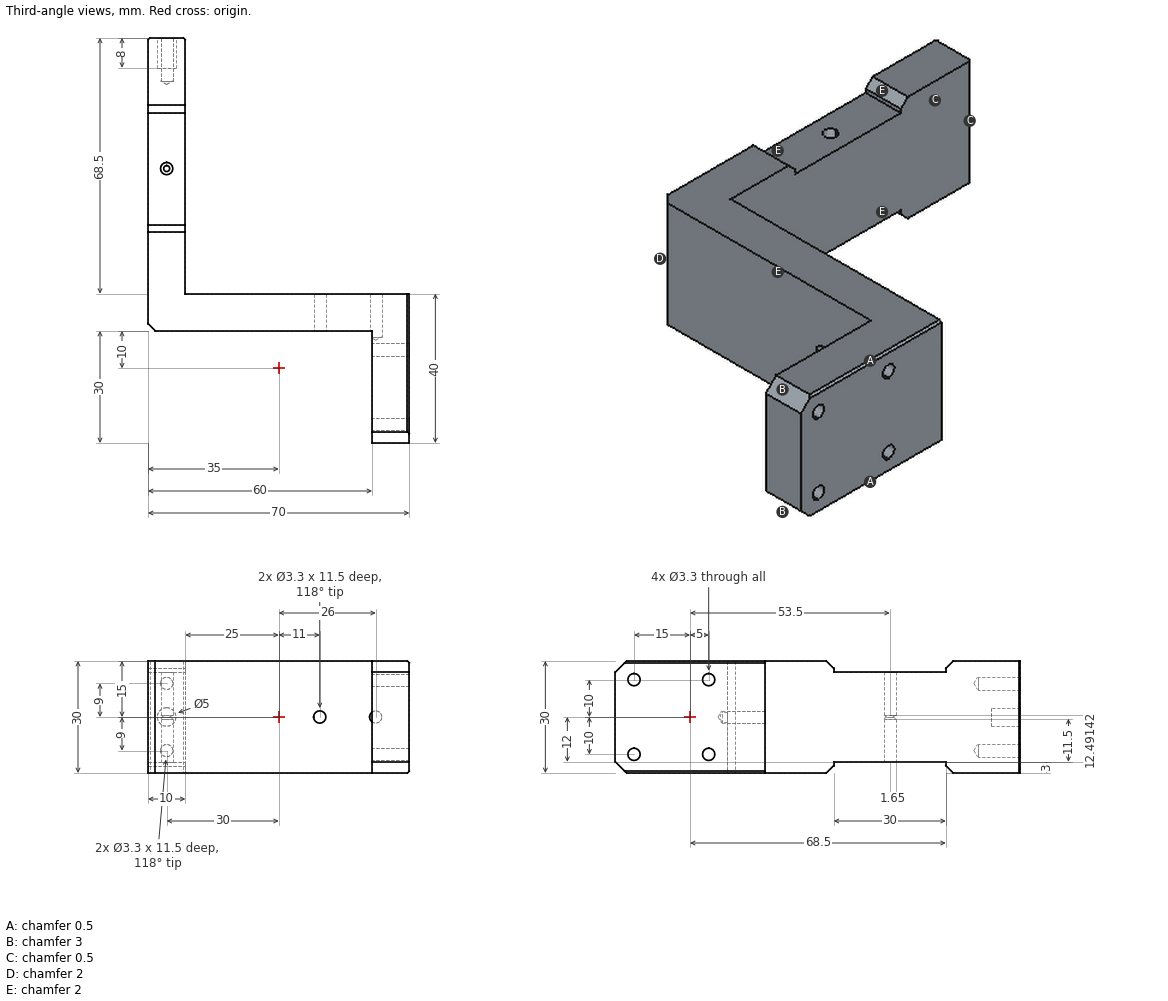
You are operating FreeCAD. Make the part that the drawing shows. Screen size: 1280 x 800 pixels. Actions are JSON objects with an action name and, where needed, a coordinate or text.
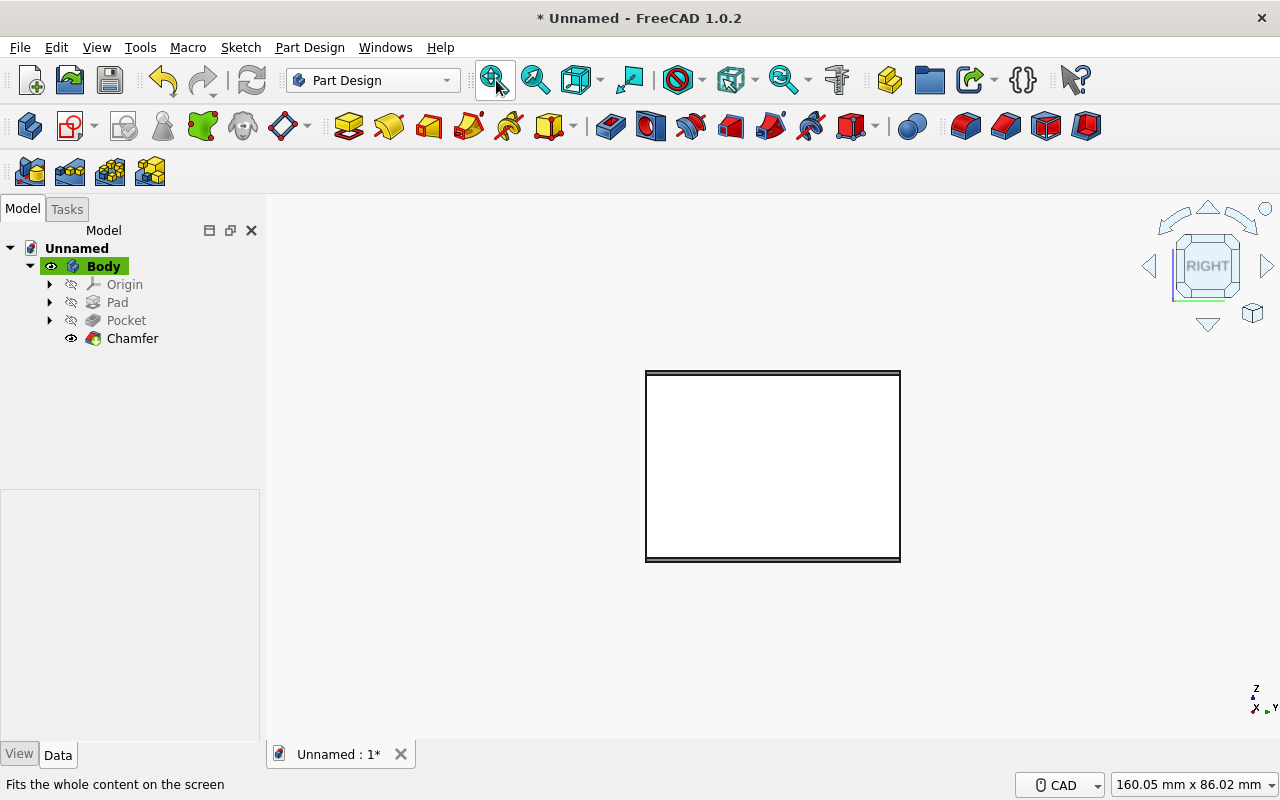
{"action": "key", "text": "v f"}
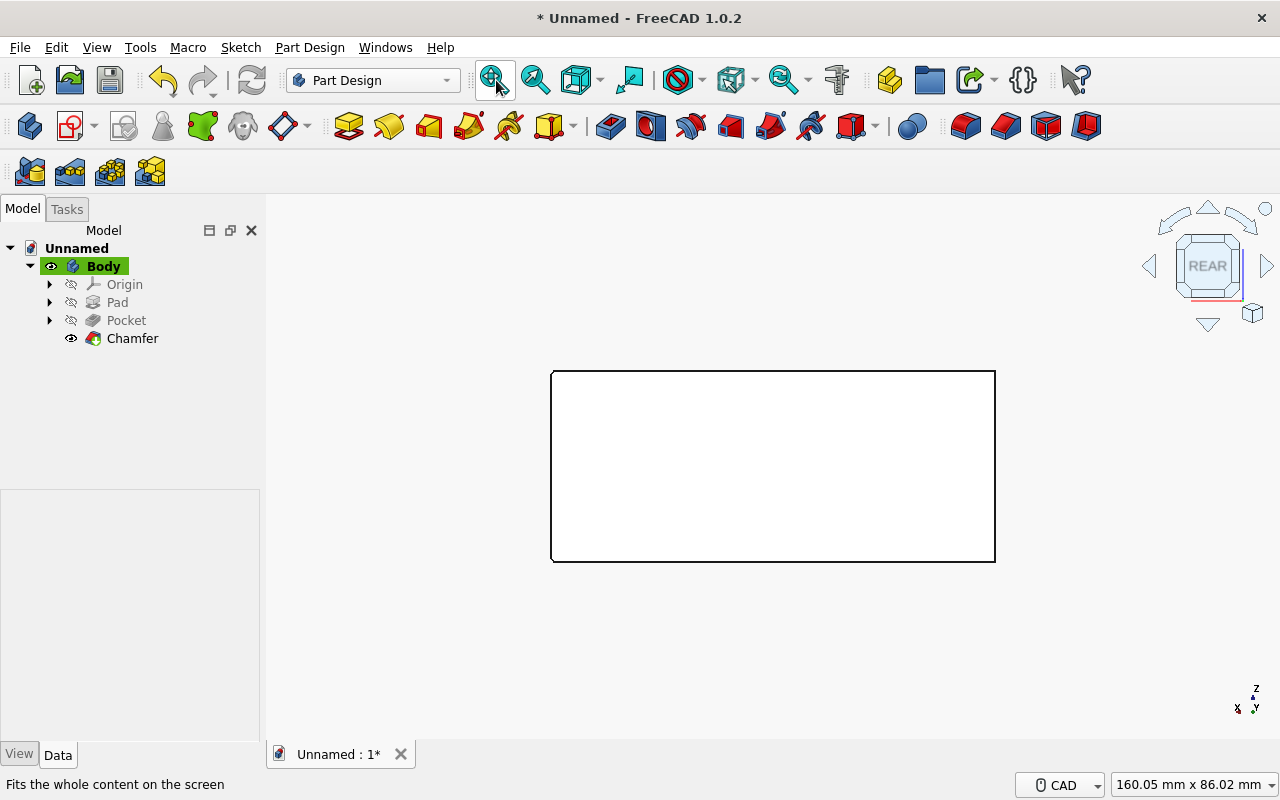
{"action": "left_click", "coordinate": [646, 466]}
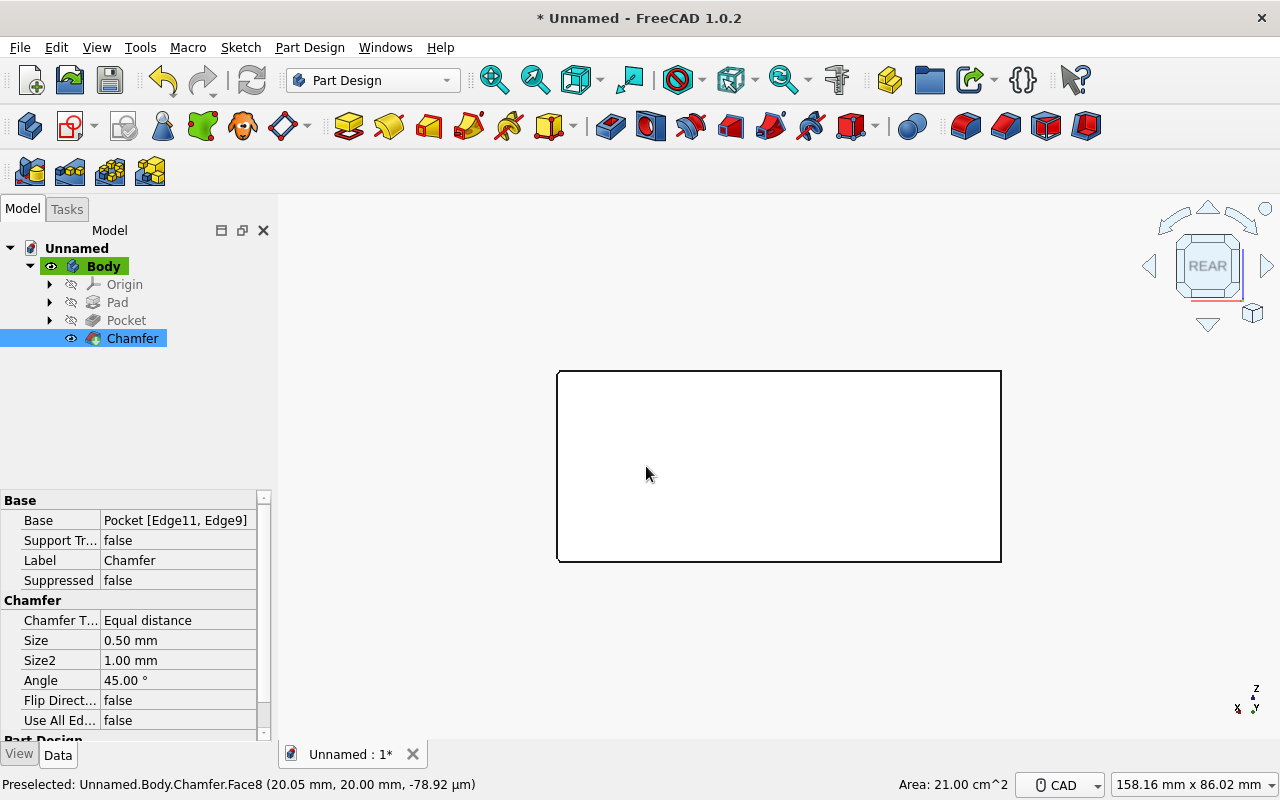
{"action": "left_click", "coordinate": [70, 126]}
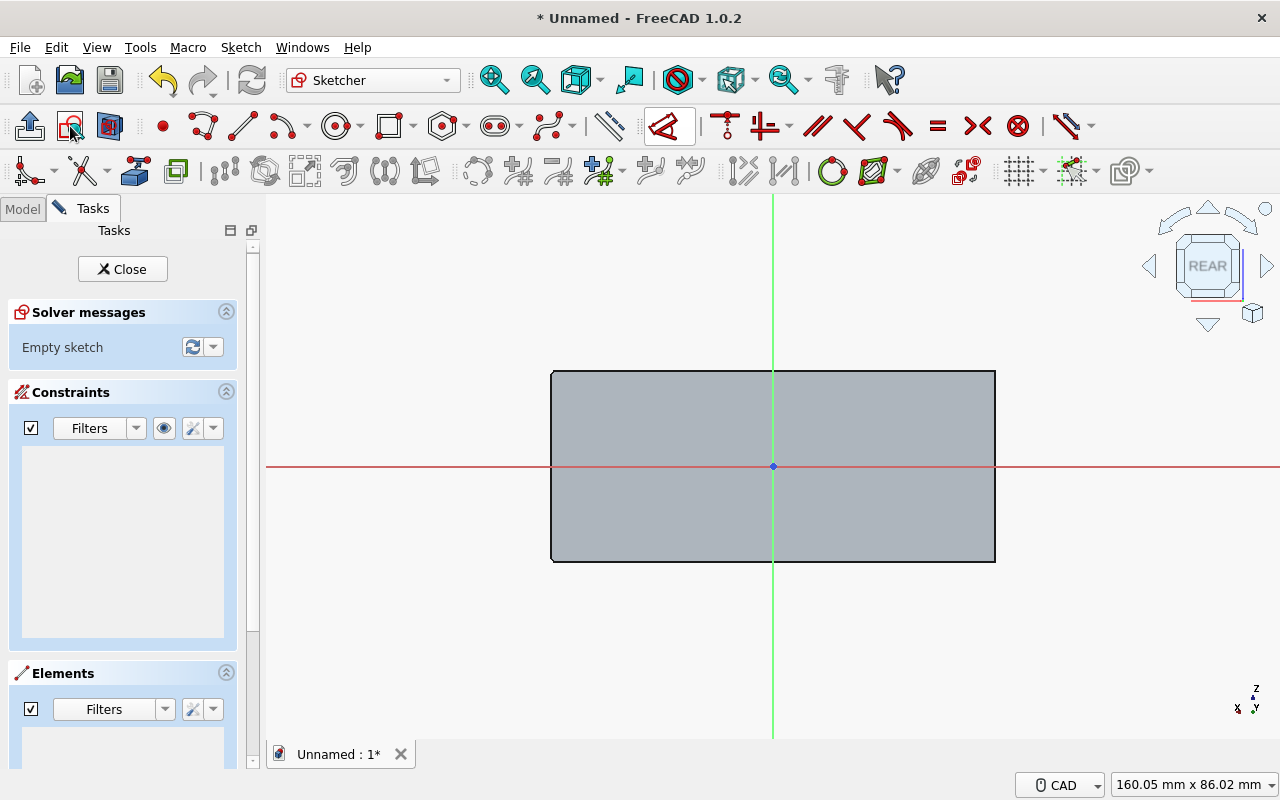
{"action": "scroll", "coordinate": [677, 466], "scroll_direction": "up", "scroll_amount": 6}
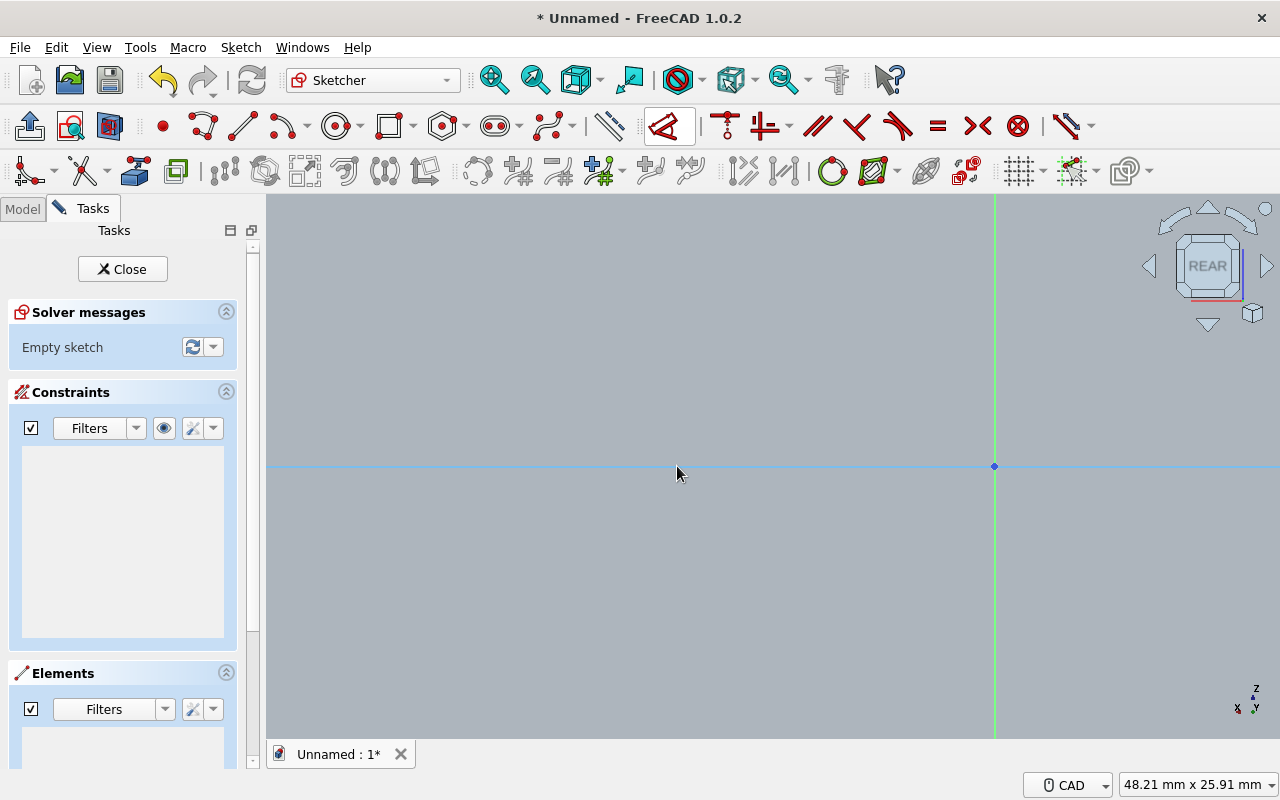
{"action": "key", "text": "g c"}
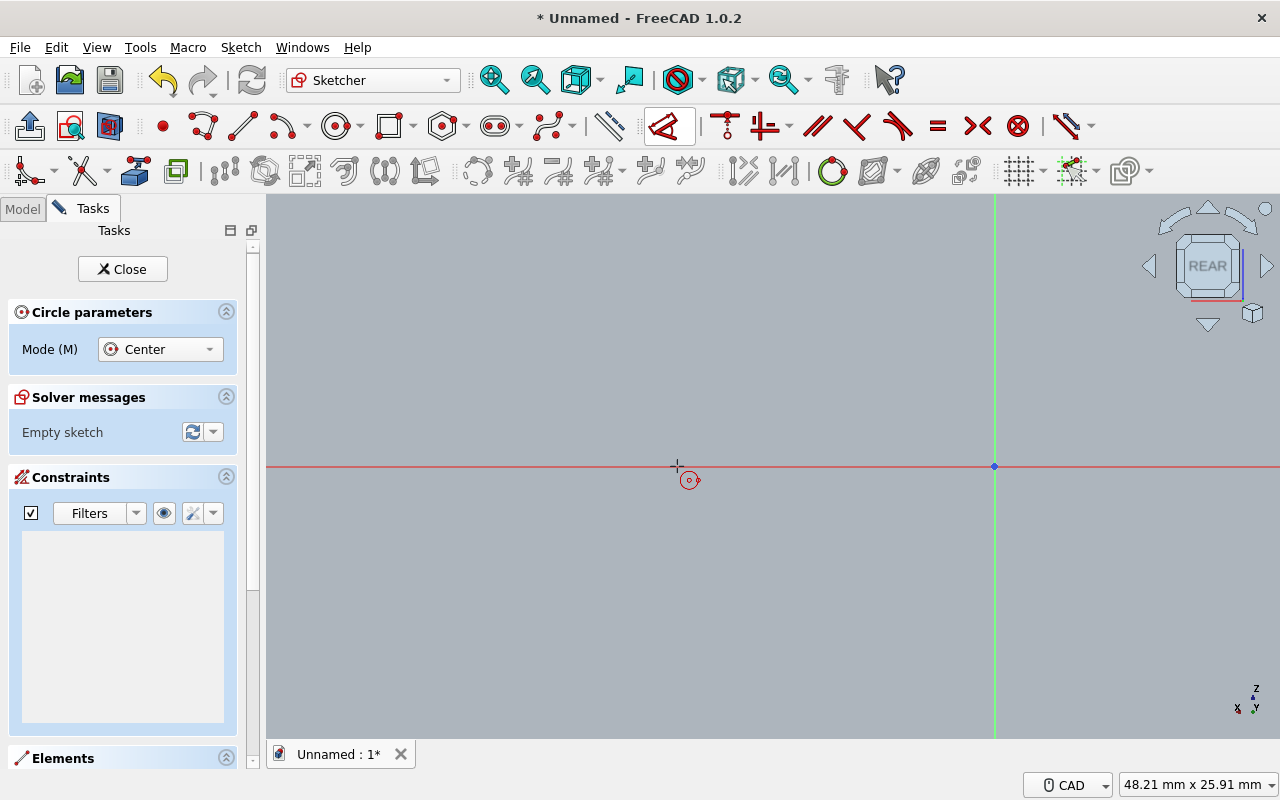
{"action": "left_click", "coordinate": [763, 466]}
{"action": "left_click", "coordinate": [788, 442]}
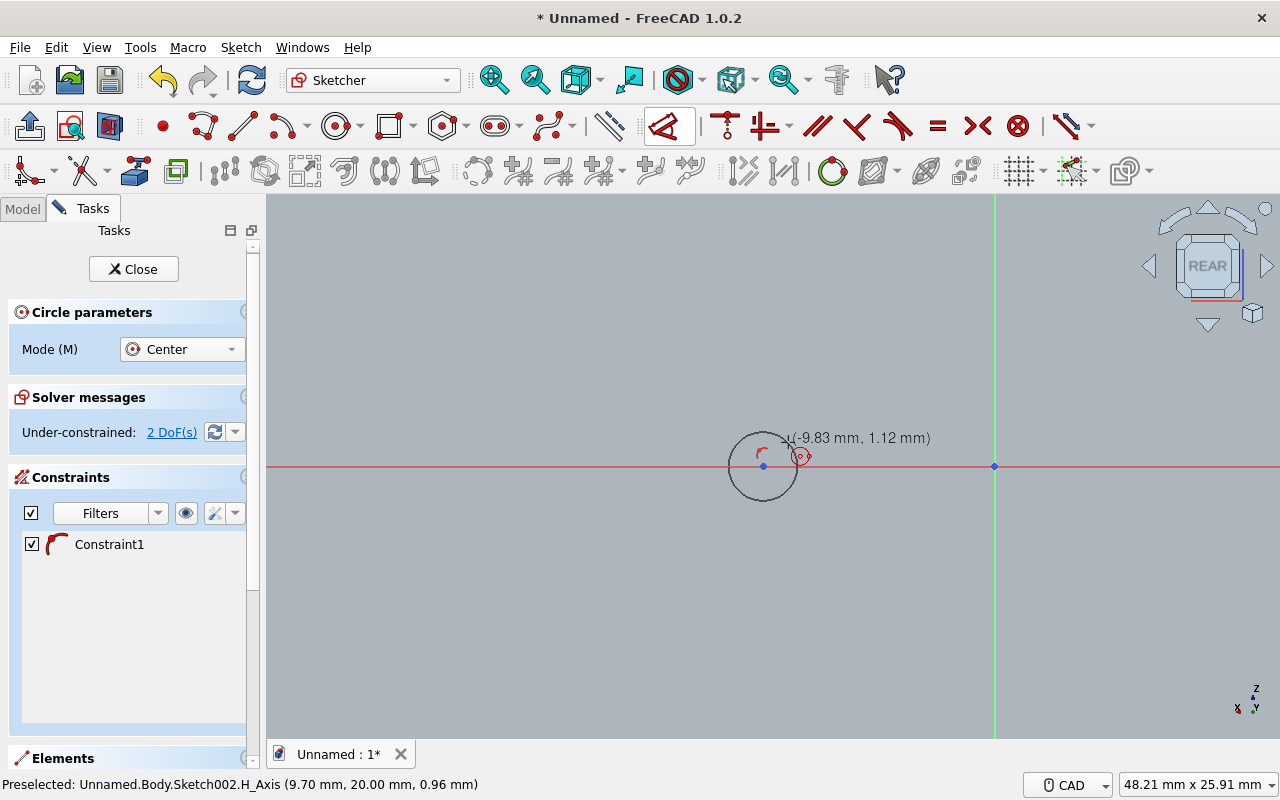
{"action": "left_click", "coordinate": [448, 466]}
{"action": "left_click", "coordinate": [472, 442]}
{"action": "key", "text": "Escape"}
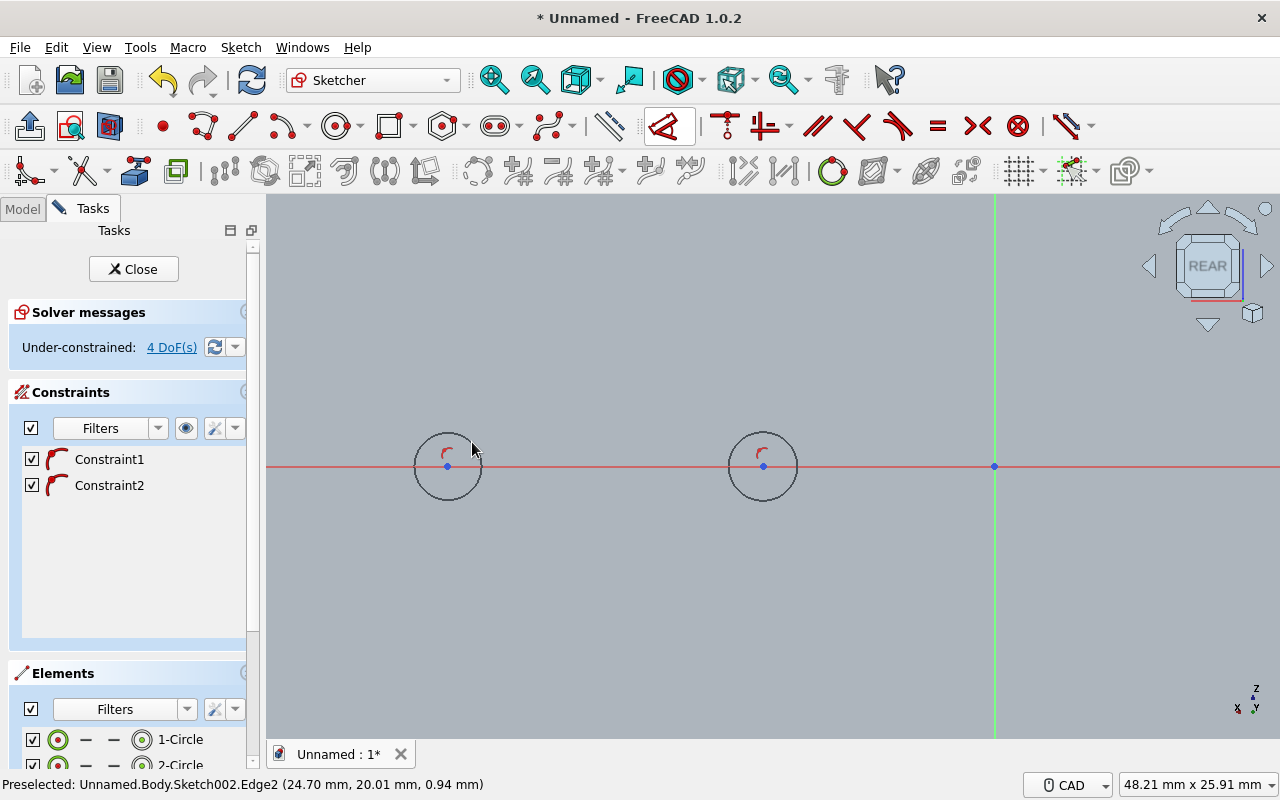
{"action": "left_click", "coordinate": [787, 442]}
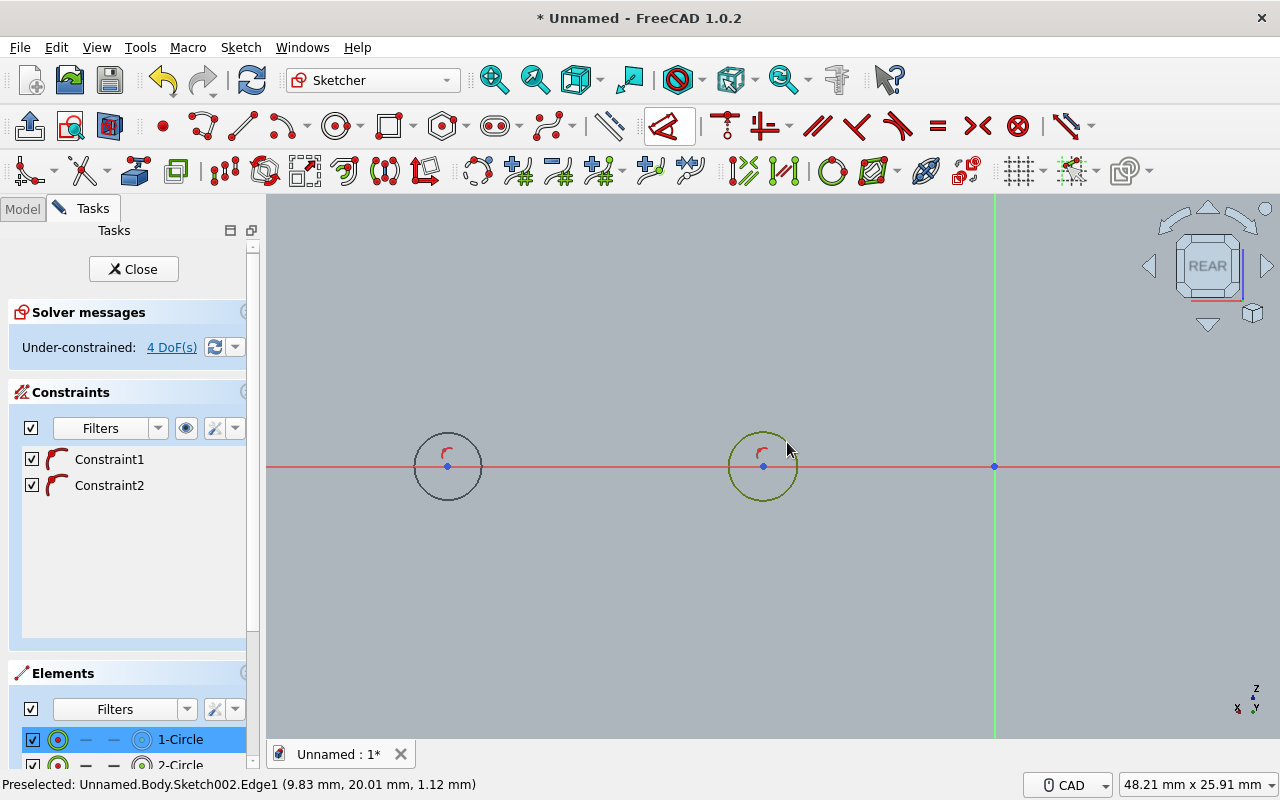
{"action": "left_click", "coordinate": [472, 443]}